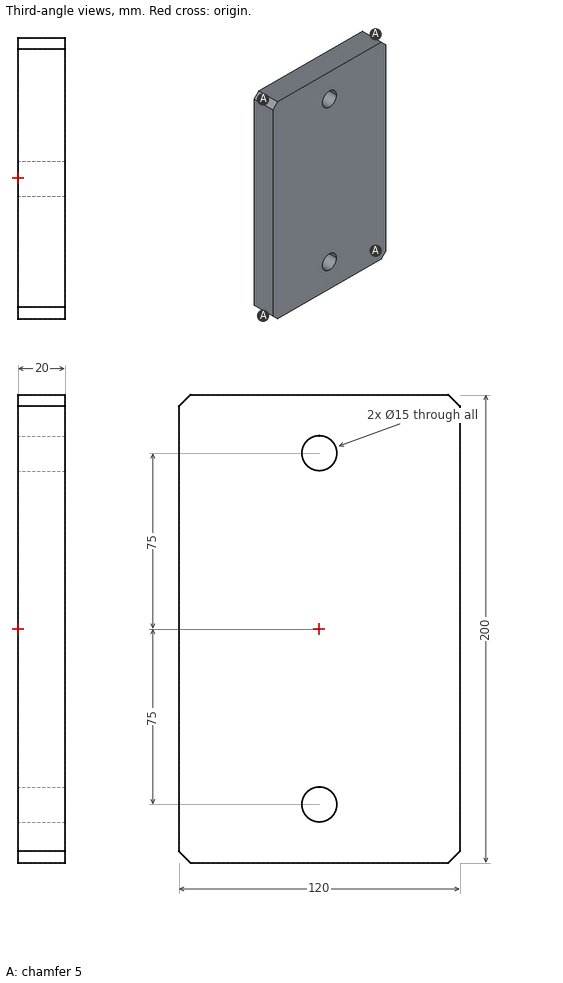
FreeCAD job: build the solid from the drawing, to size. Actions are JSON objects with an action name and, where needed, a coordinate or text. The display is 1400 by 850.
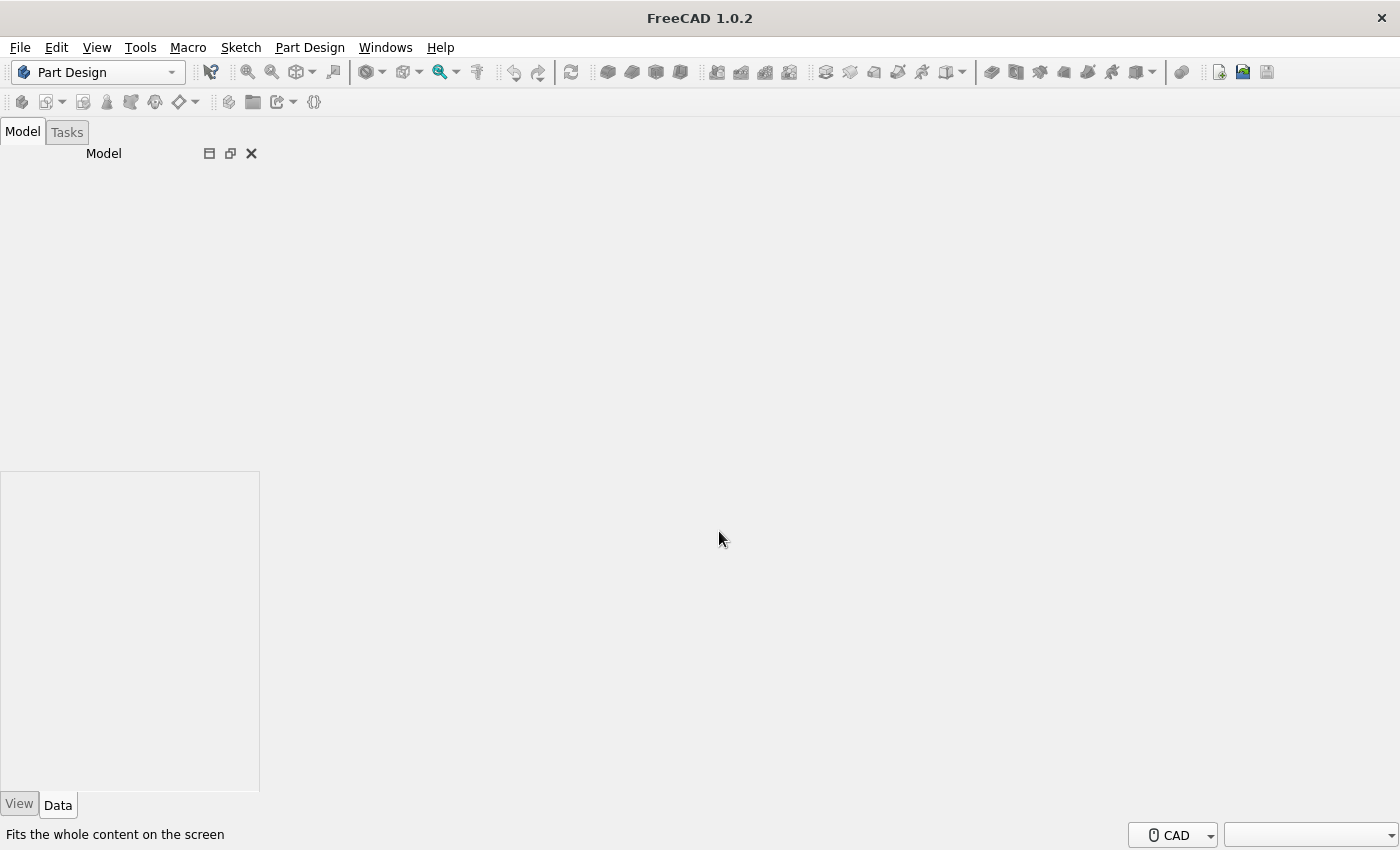
{"action": "left_click", "coordinate": [1220, 72]}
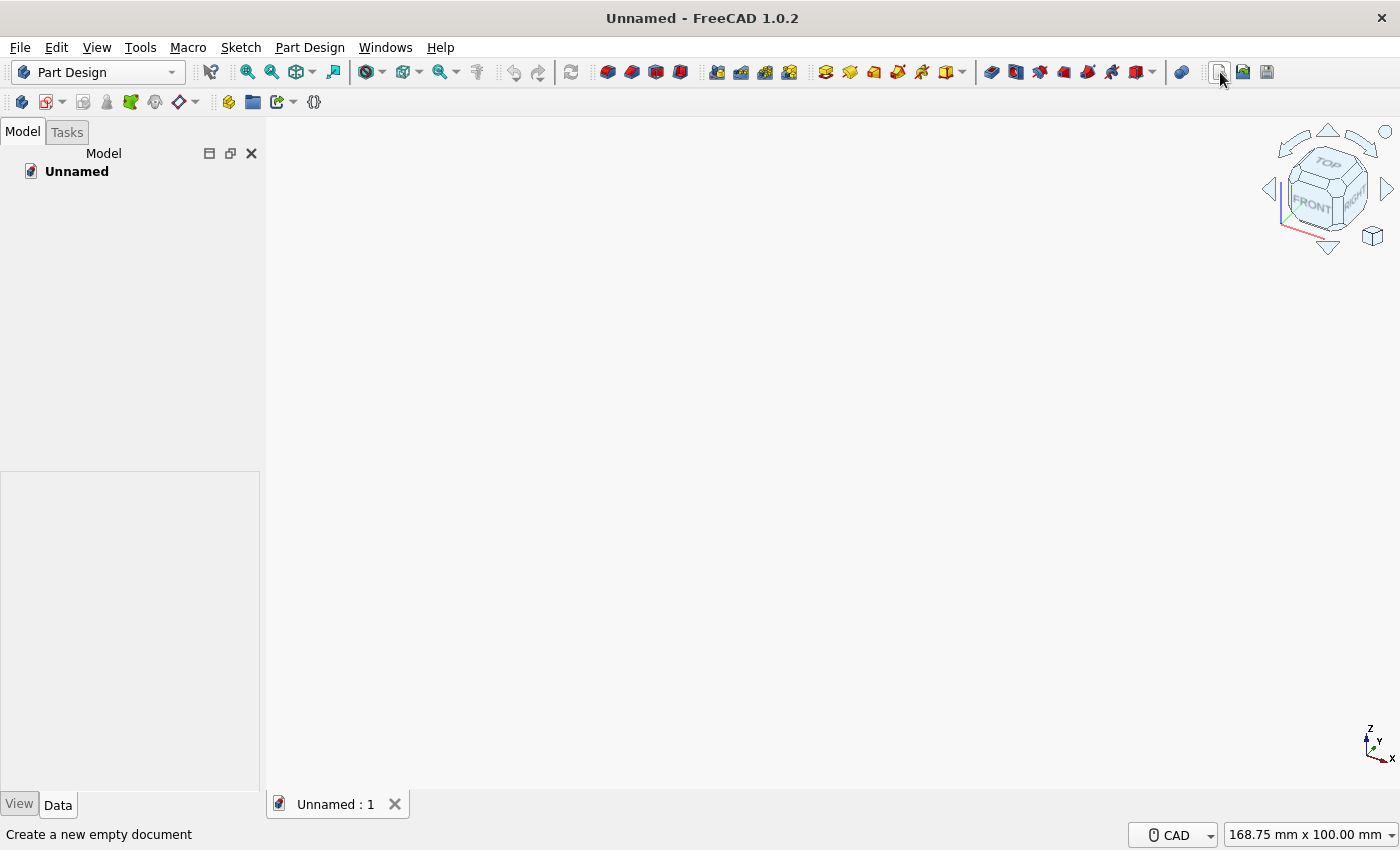
{"action": "left_click", "coordinate": [46, 102]}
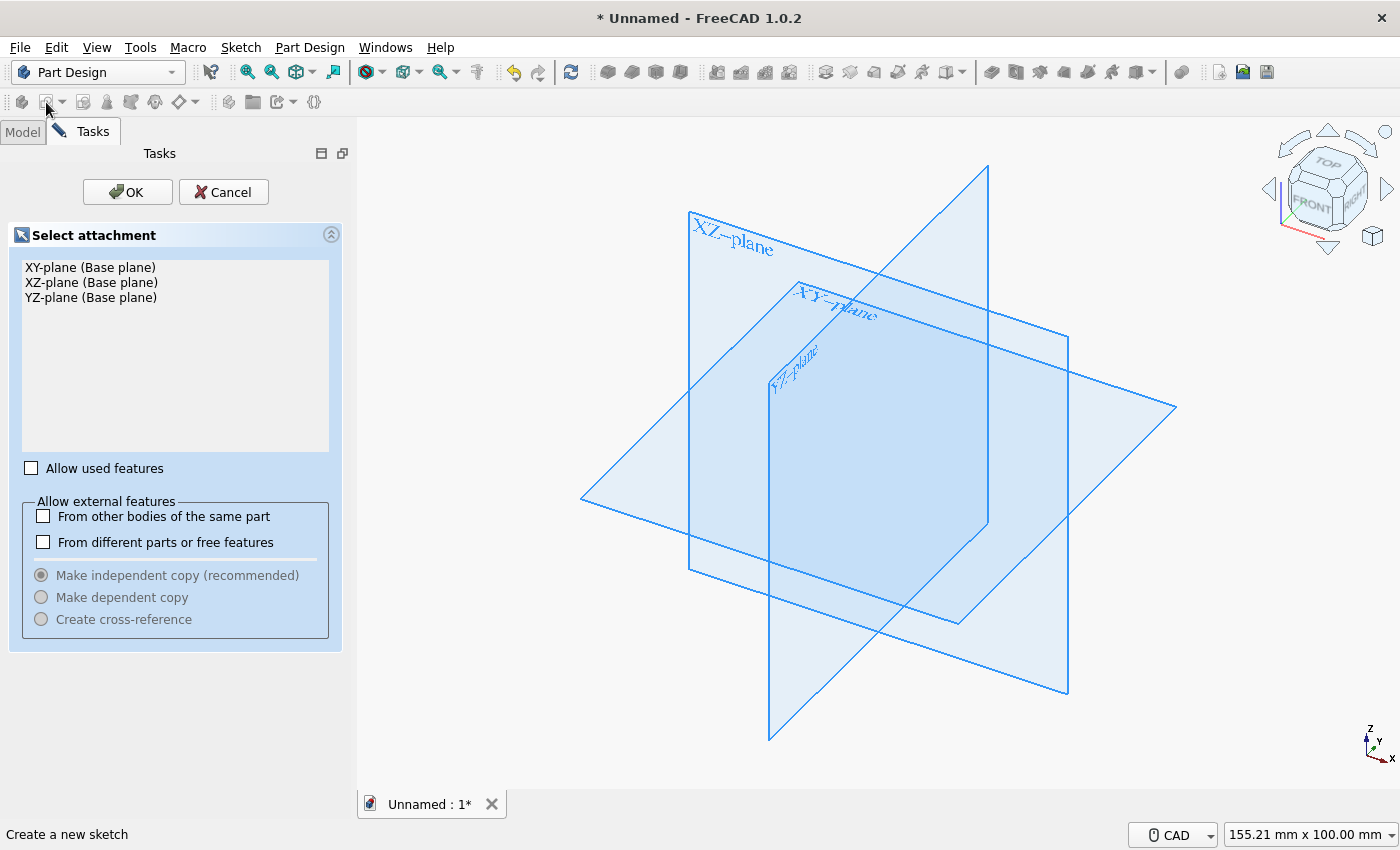
{"action": "left_click", "coordinate": [82, 298]}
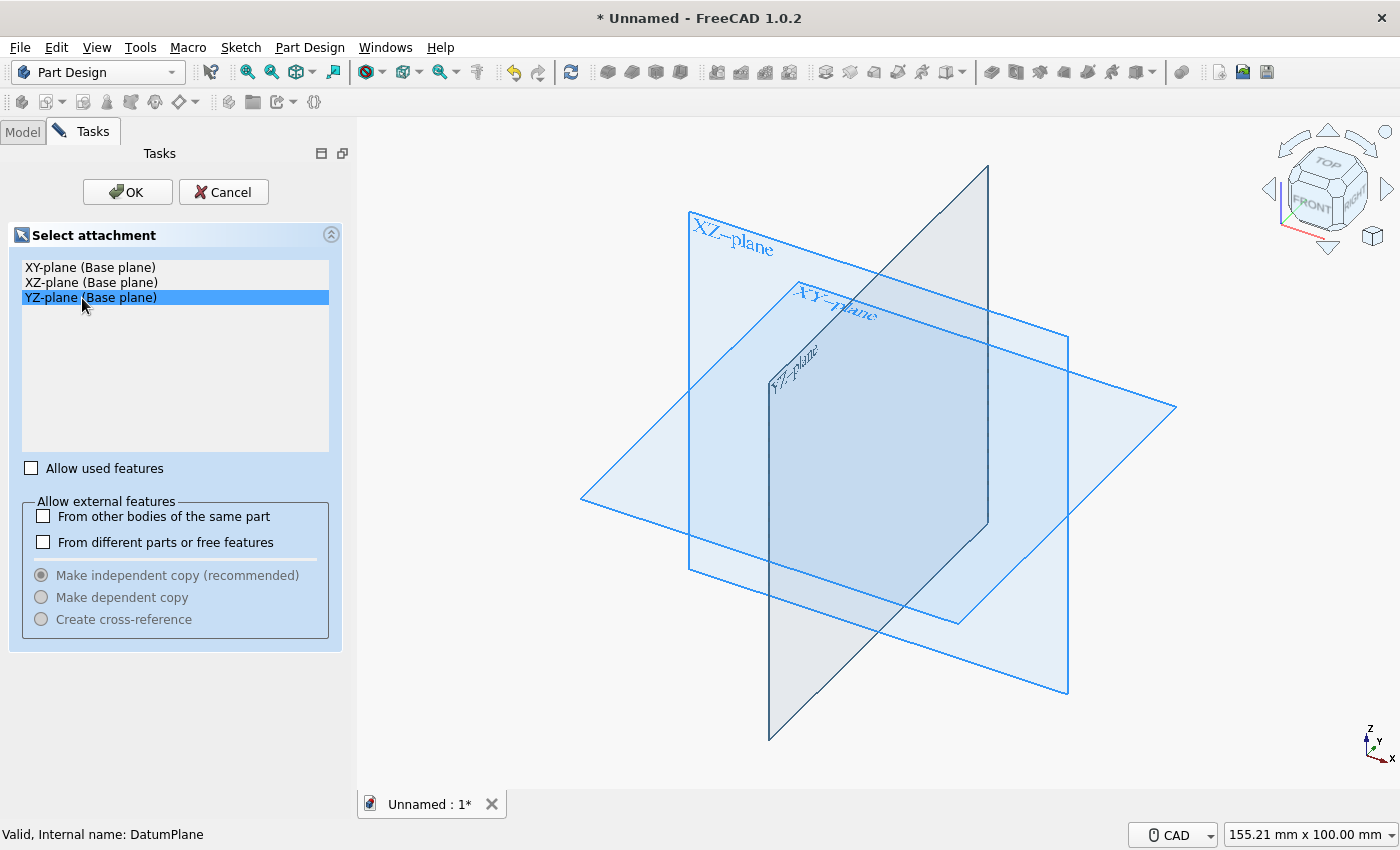
{"action": "left_click", "coordinate": [128, 192]}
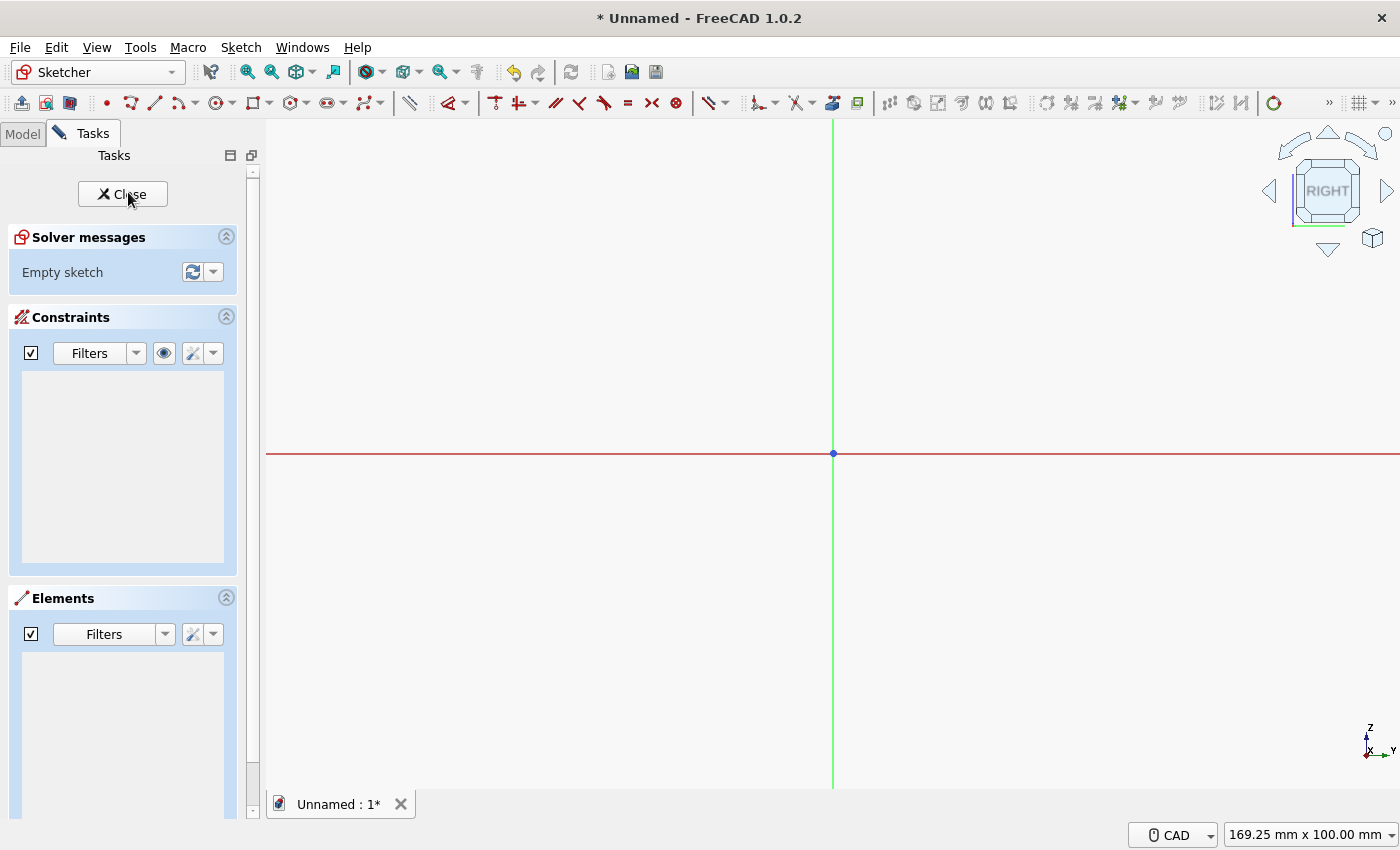
{"action": "scroll", "coordinate": [735, 454], "scroll_direction": "down", "scroll_amount": 6}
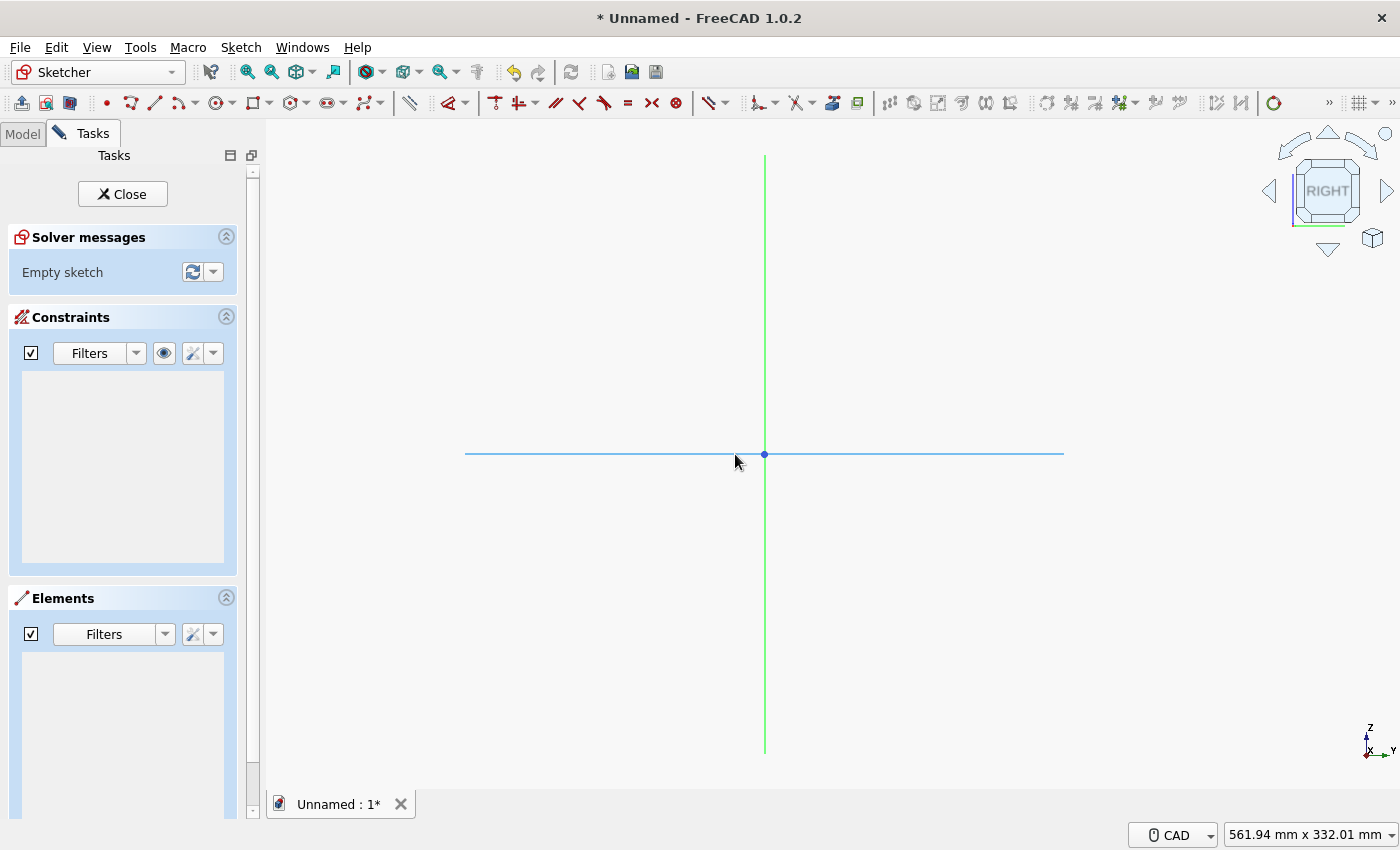
{"action": "left_click", "coordinate": [272, 104]}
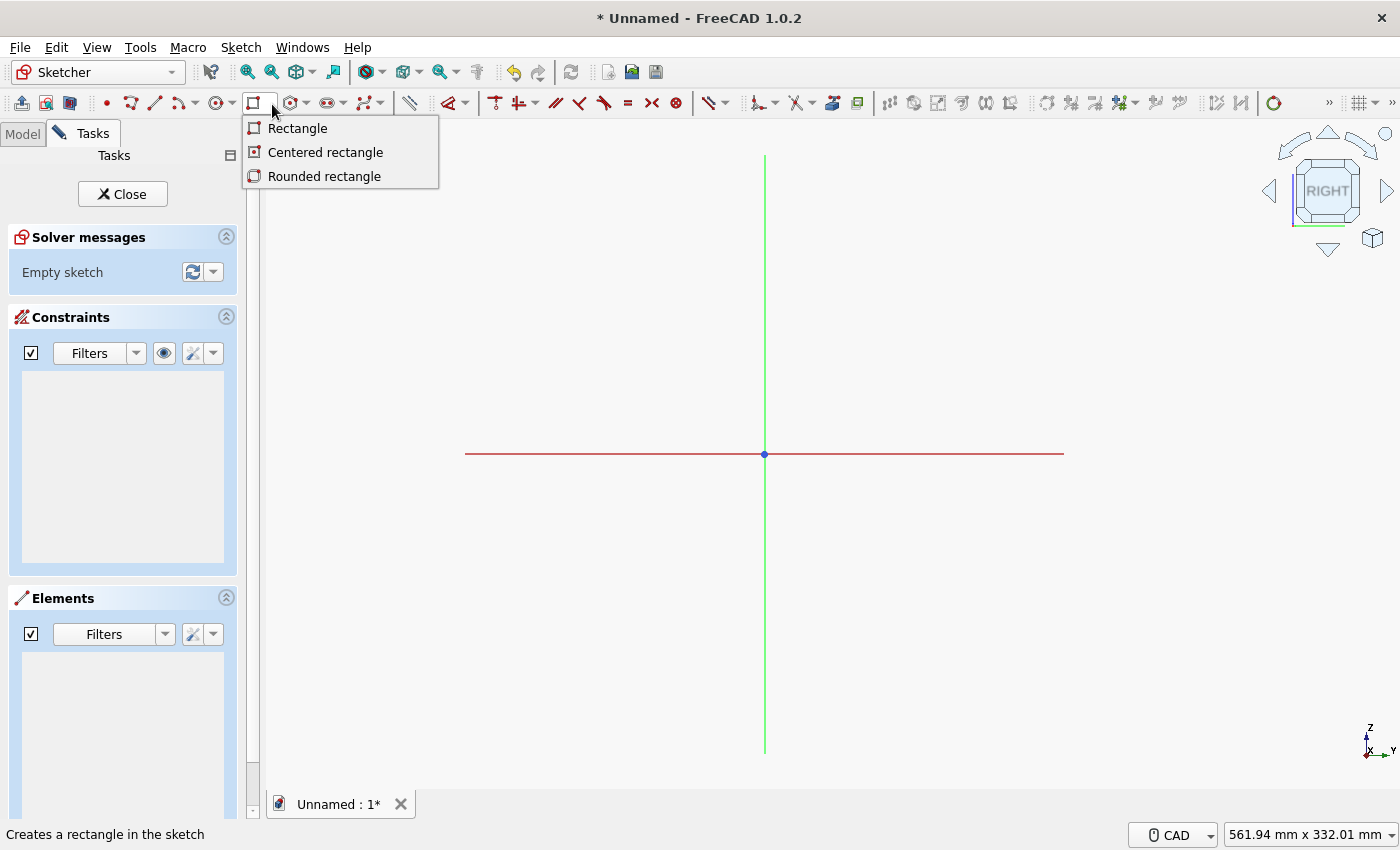
{"action": "left_click", "coordinate": [340, 152]}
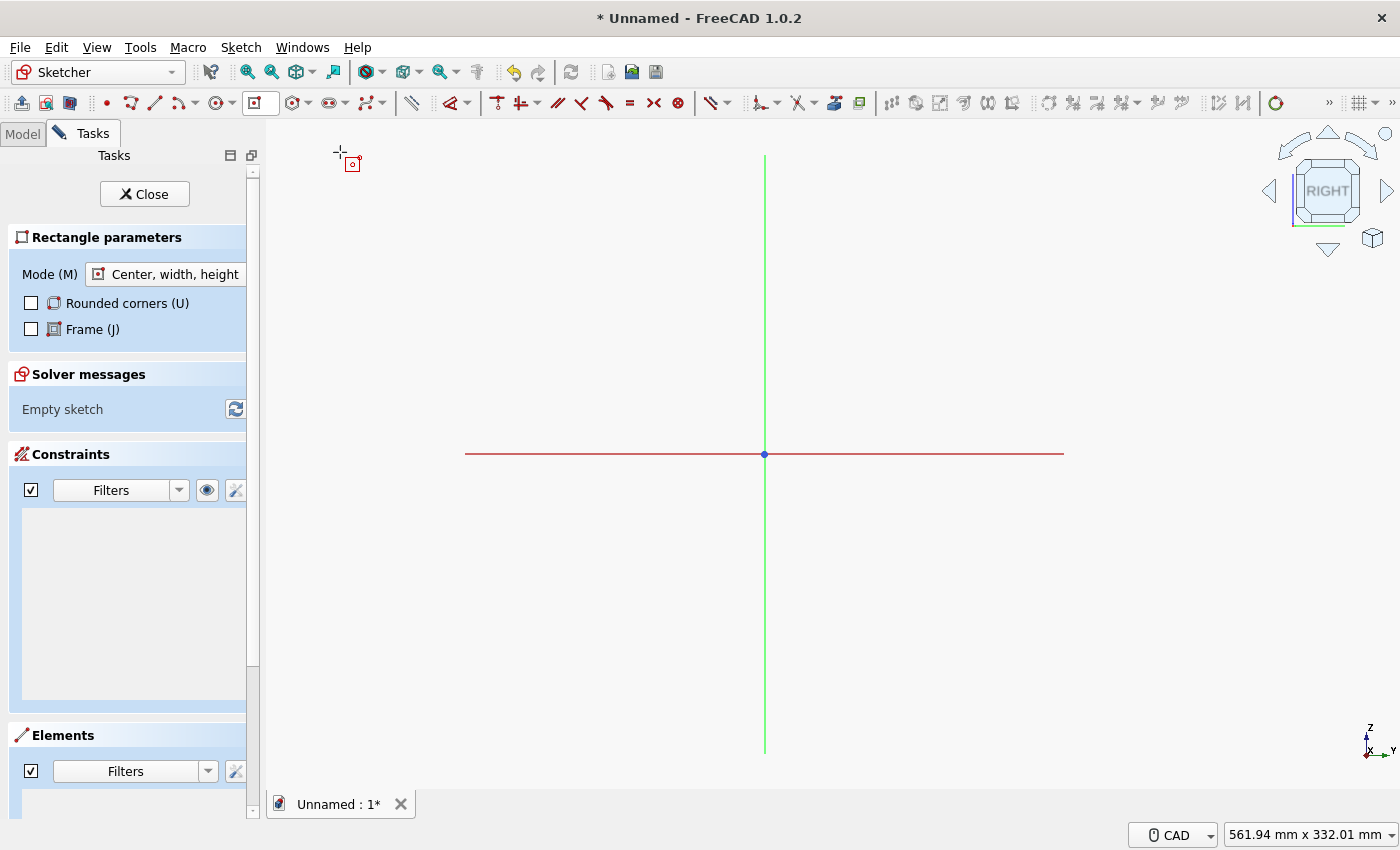
{"action": "left_click", "coordinate": [765, 454]}
{"action": "left_click", "coordinate": [886, 253]}
{"action": "key", "text": "Escape"}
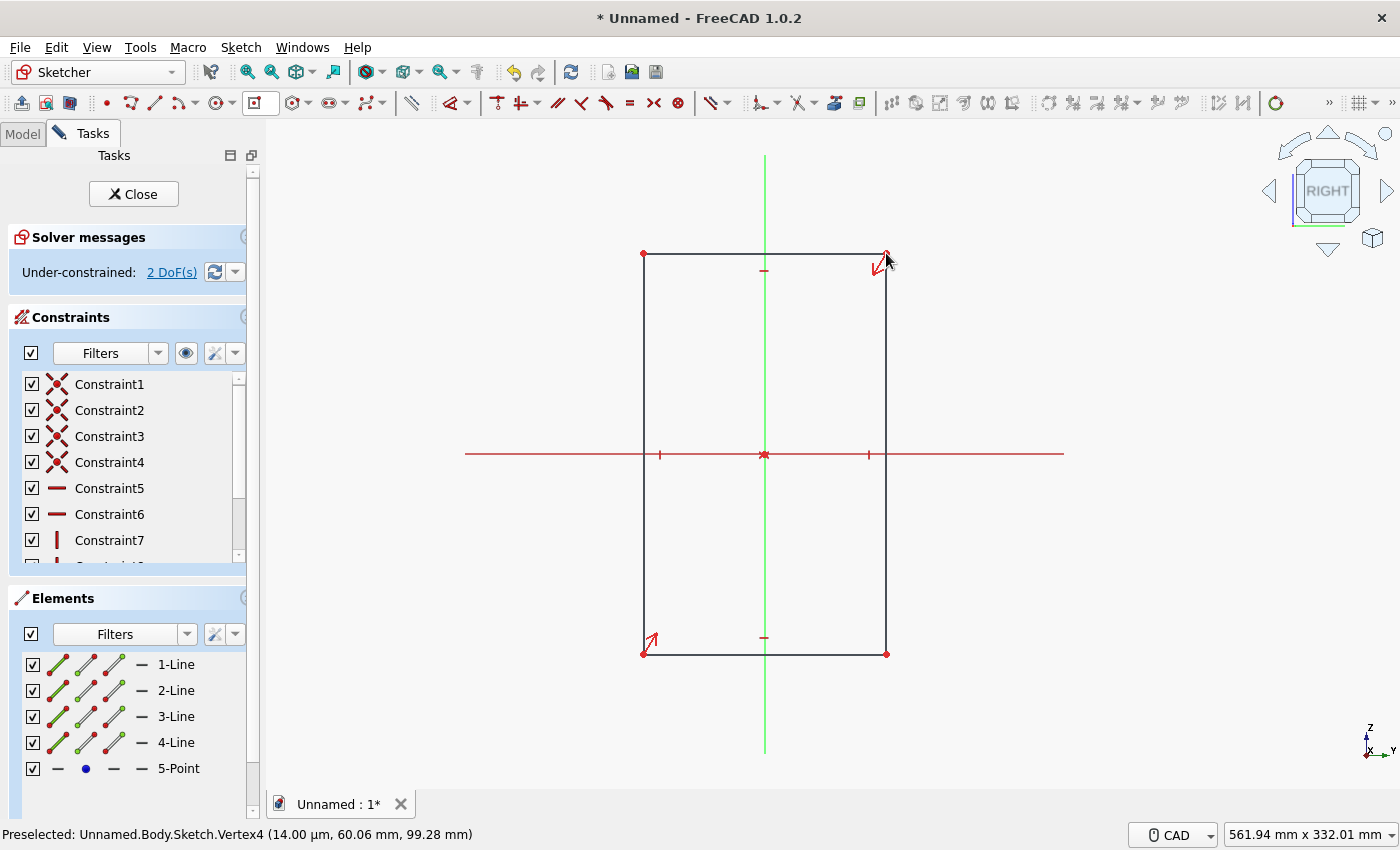
{"action": "key", "text": "d"}